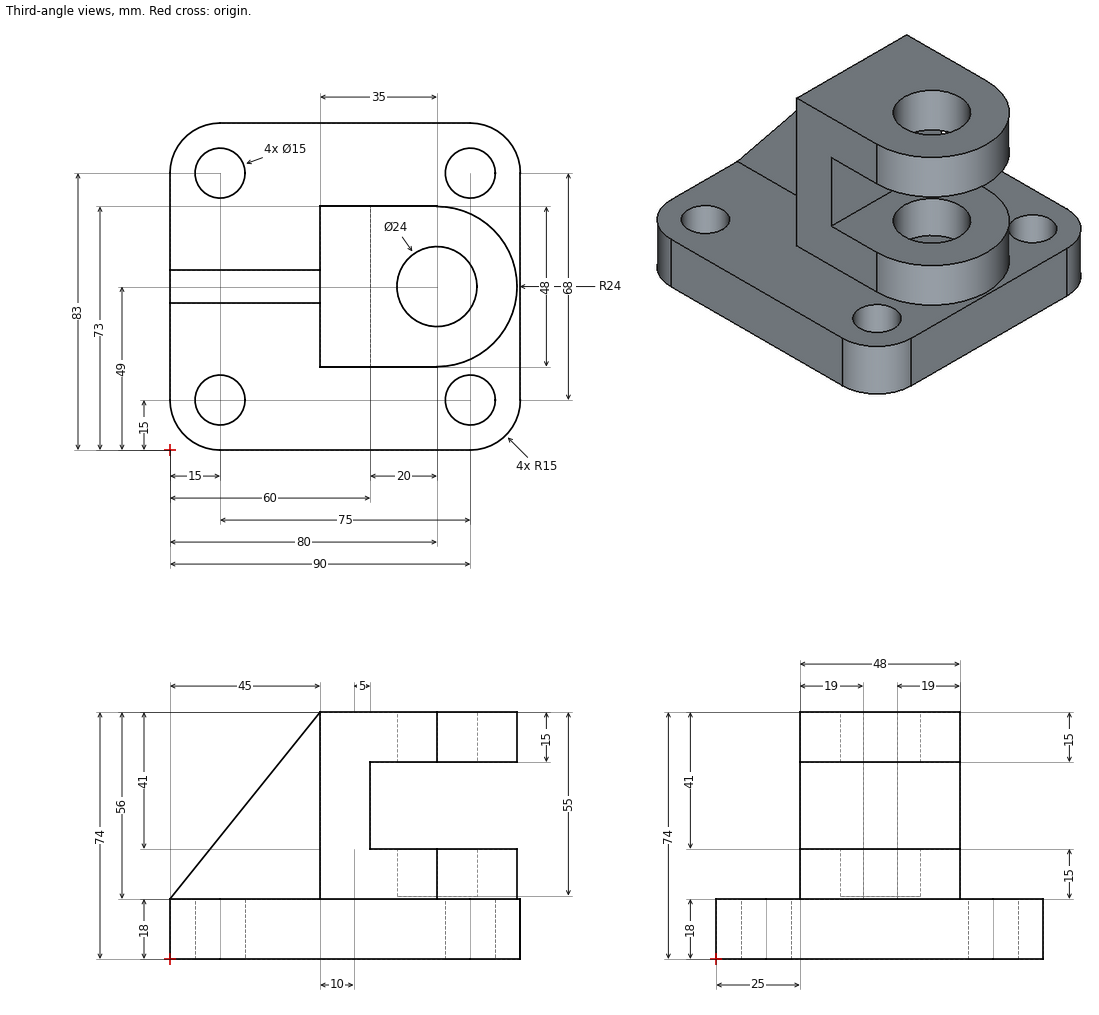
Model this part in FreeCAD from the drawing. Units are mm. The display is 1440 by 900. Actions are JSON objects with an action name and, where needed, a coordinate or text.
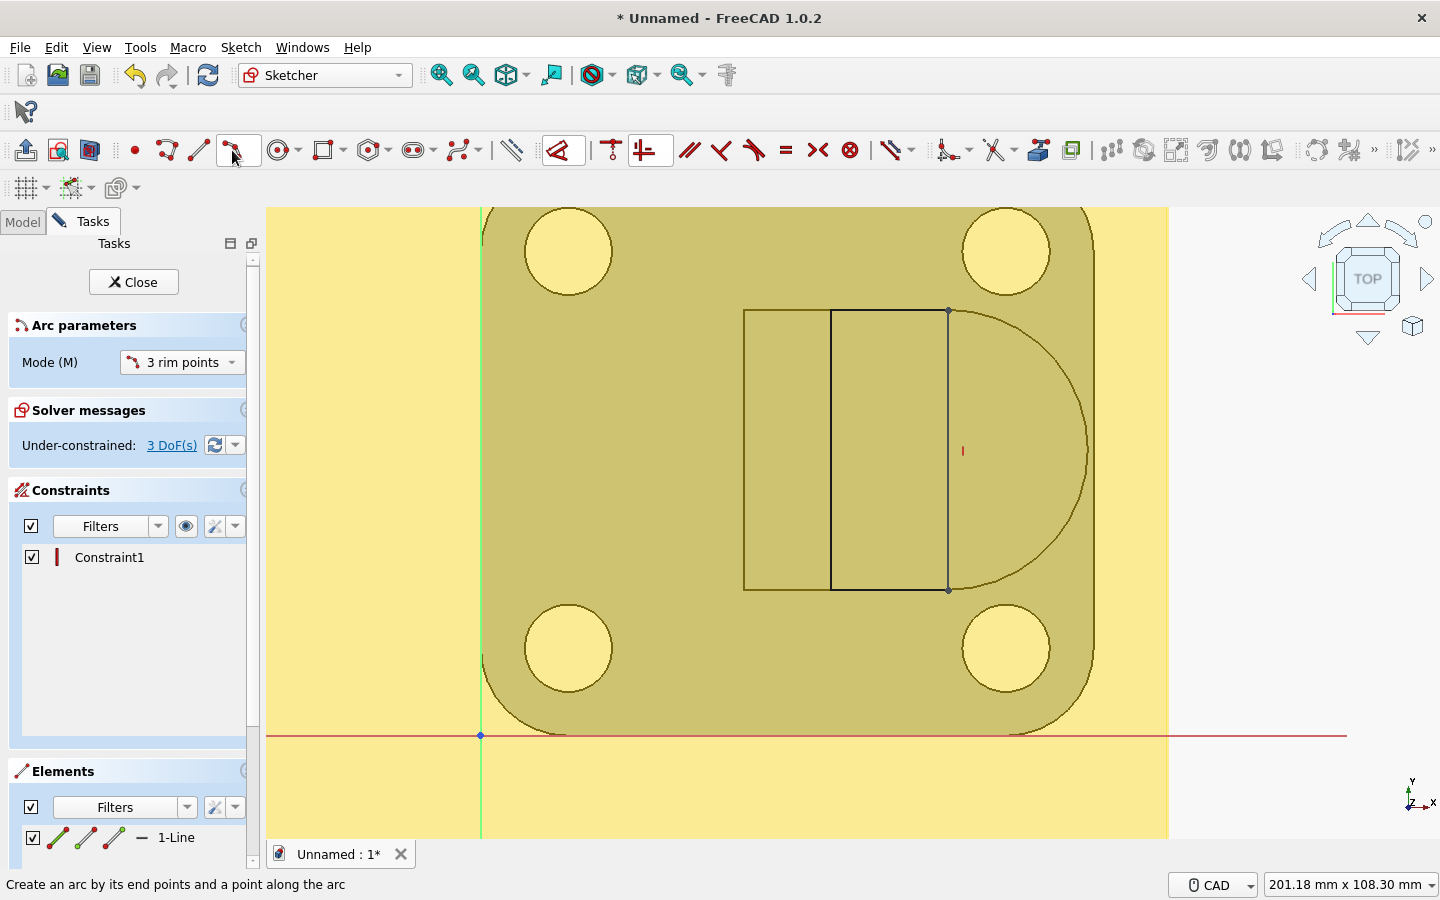
{"action": "left_click", "coordinate": [948, 591]}
{"action": "left_click", "coordinate": [948, 311]}
{"action": "left_click", "coordinate": [1088, 450]}
{"action": "key", "text": "Escape"}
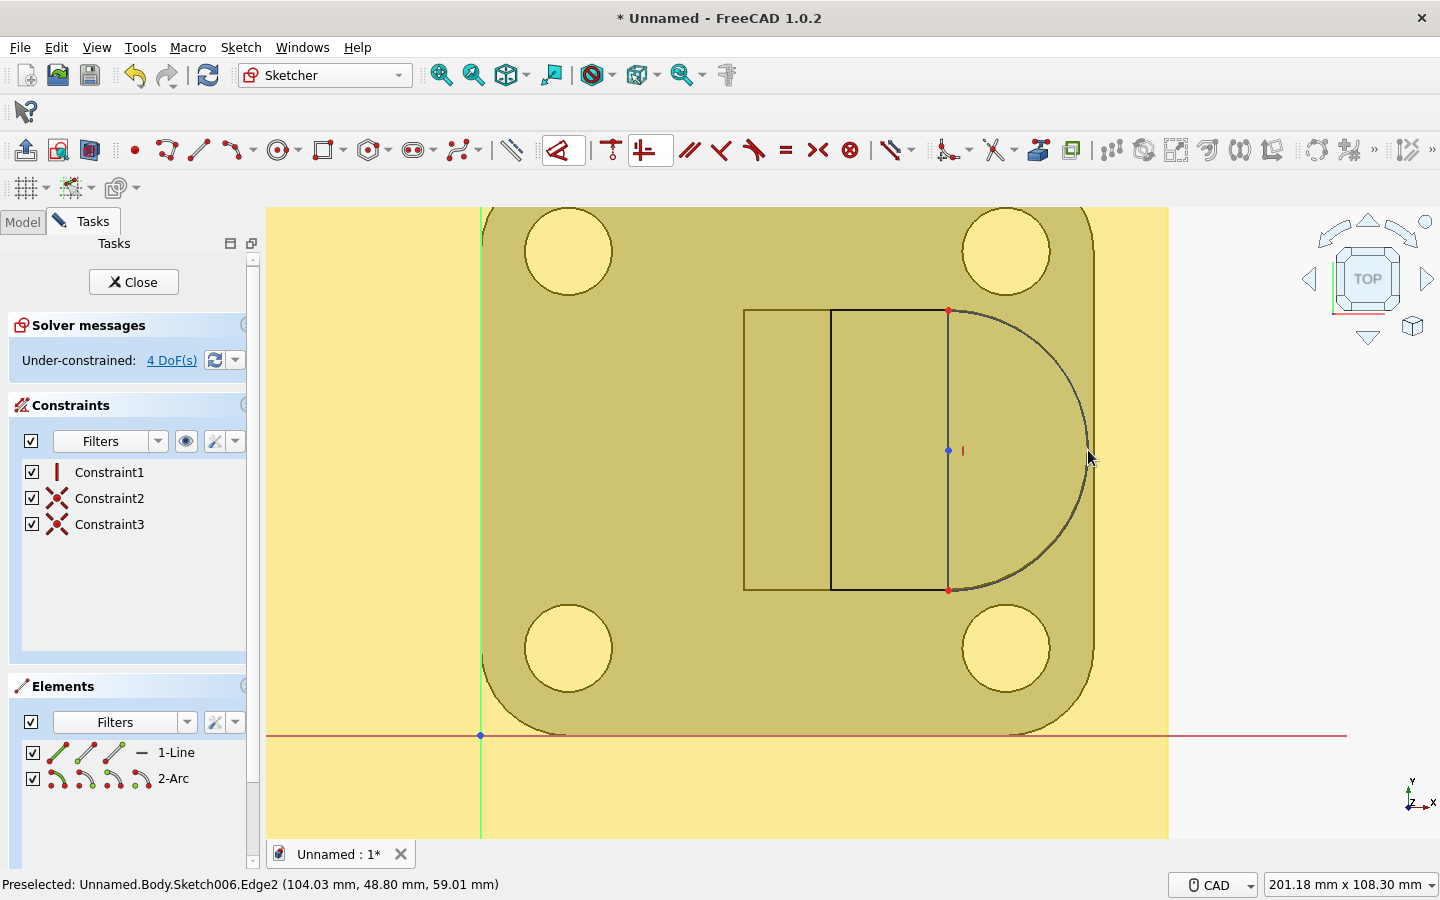
{"action": "left_click", "coordinate": [1061, 533]}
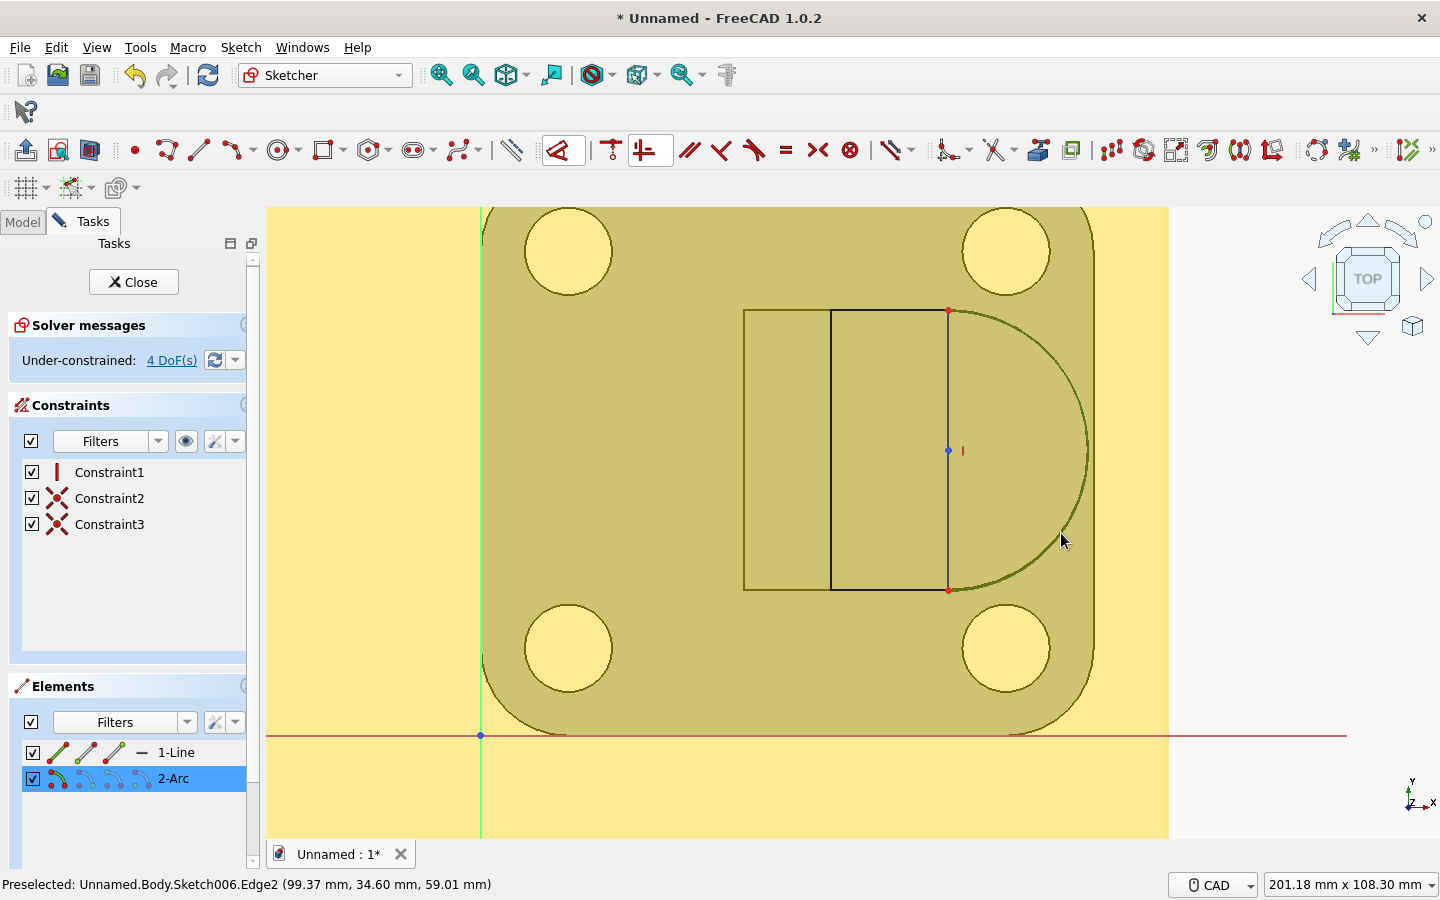
{"action": "left_click", "coordinate": [580, 150]}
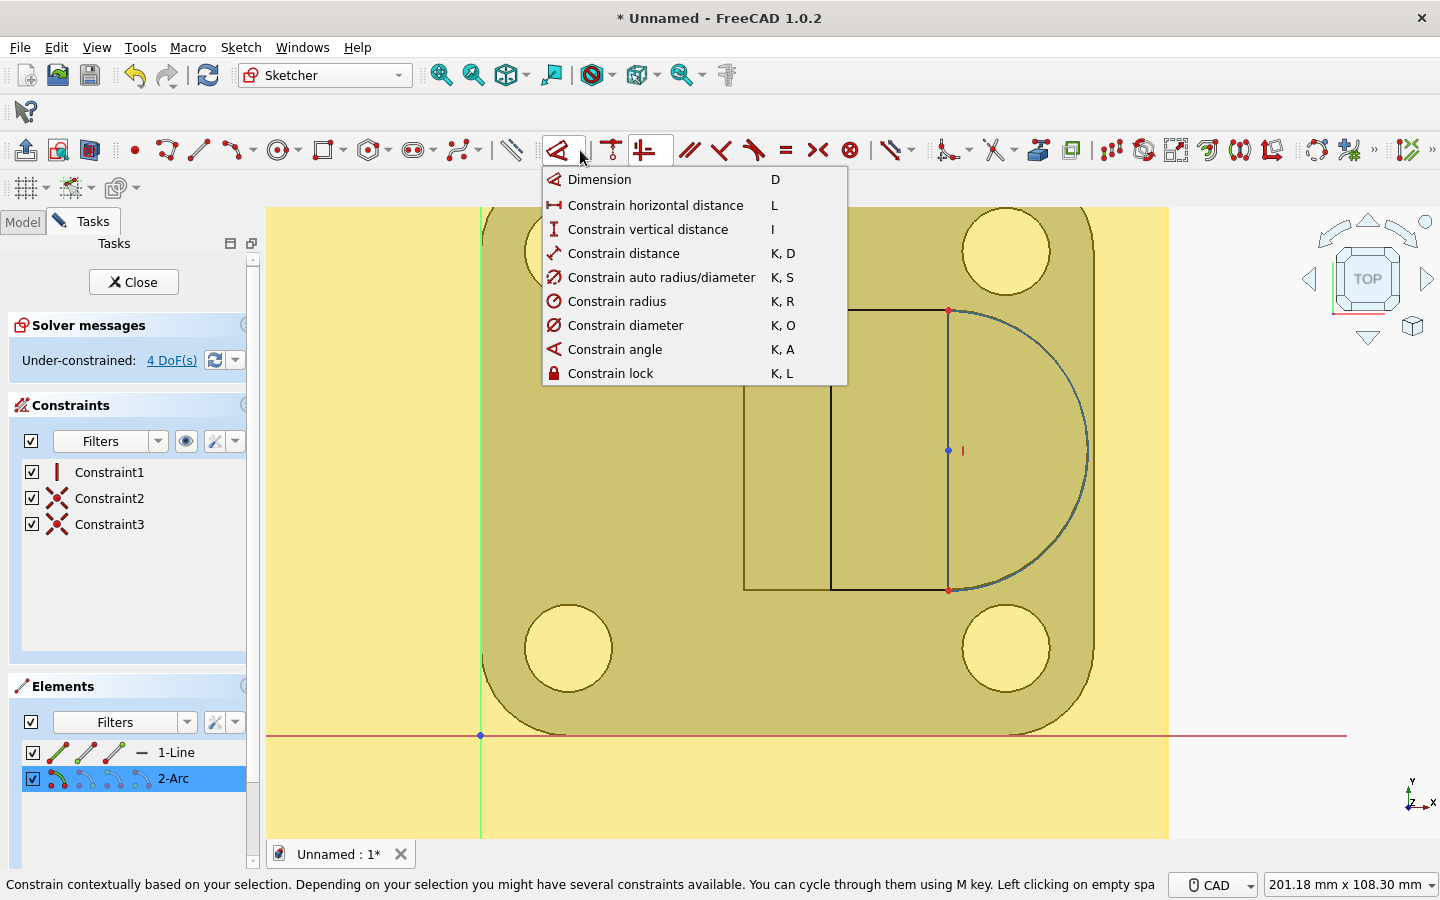
{"action": "left_click", "coordinate": [695, 301]}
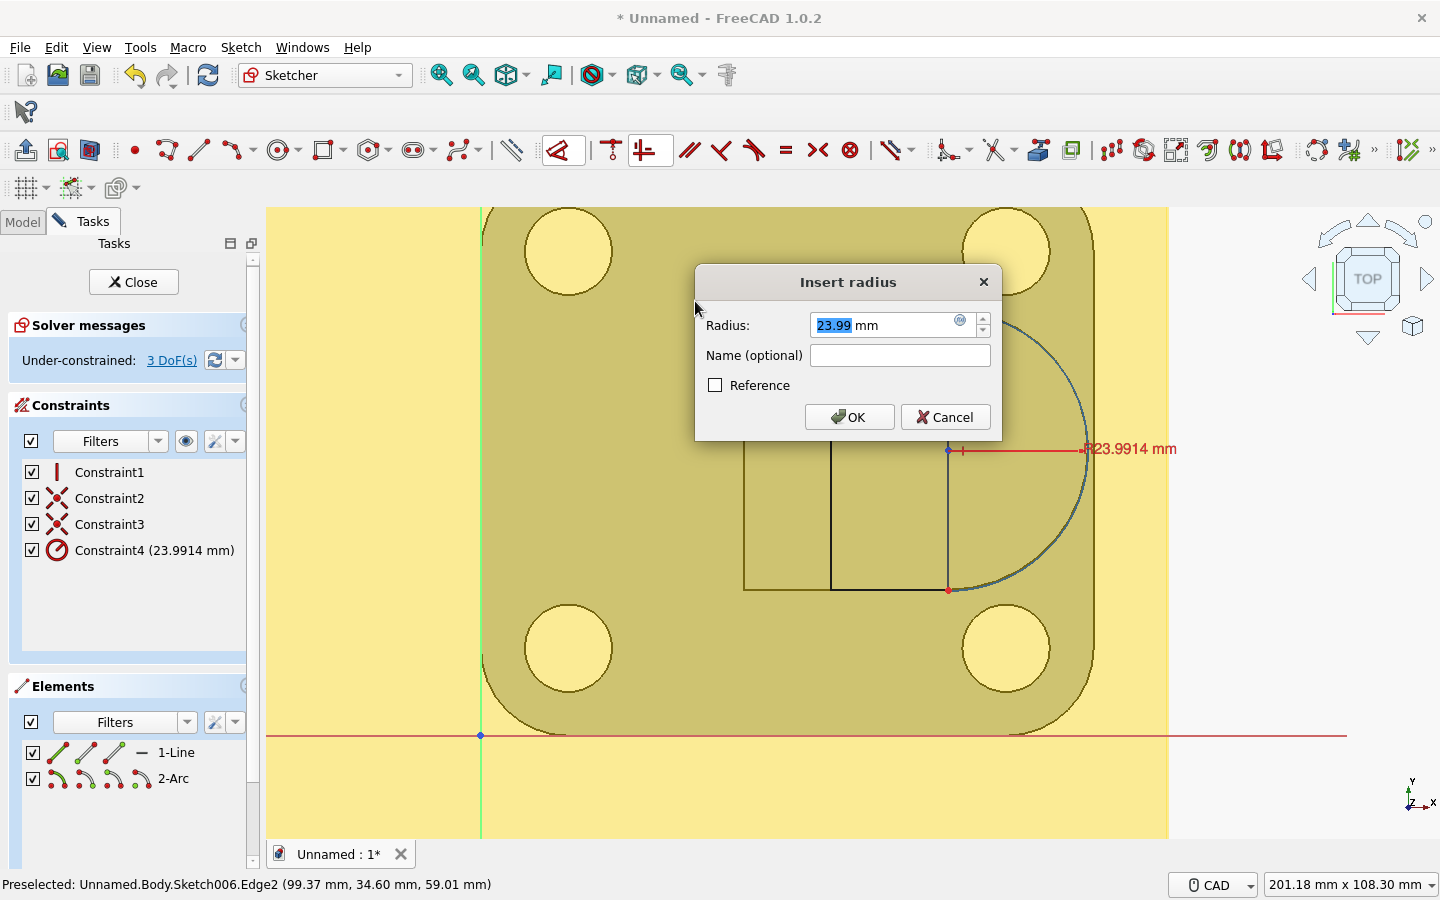
{"action": "type", "text": "24"}
{"action": "key", "text": "Return"}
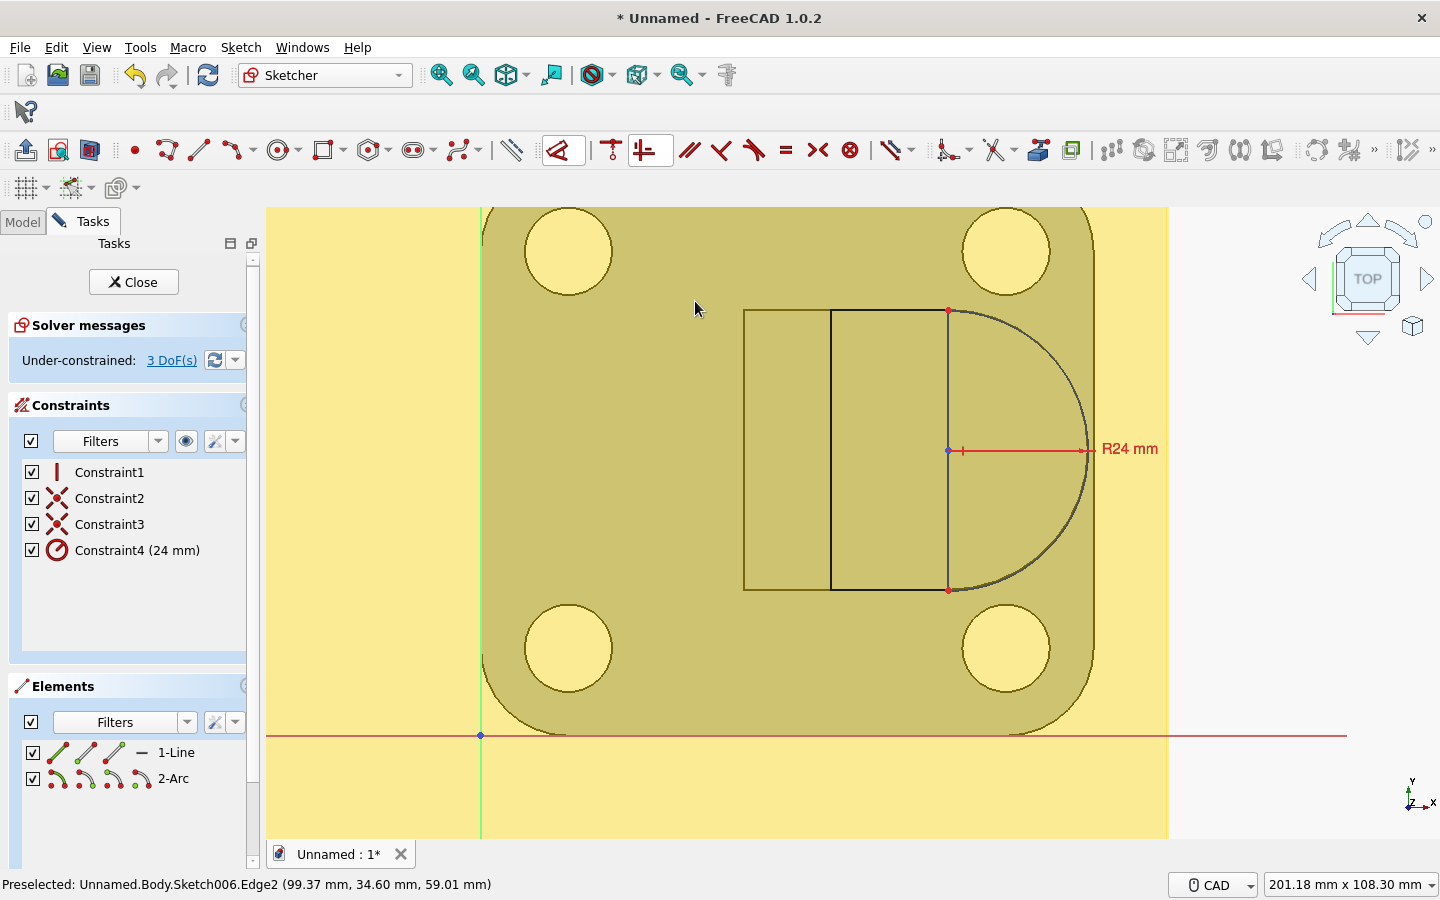
{"action": "left_click", "coordinate": [948, 311]}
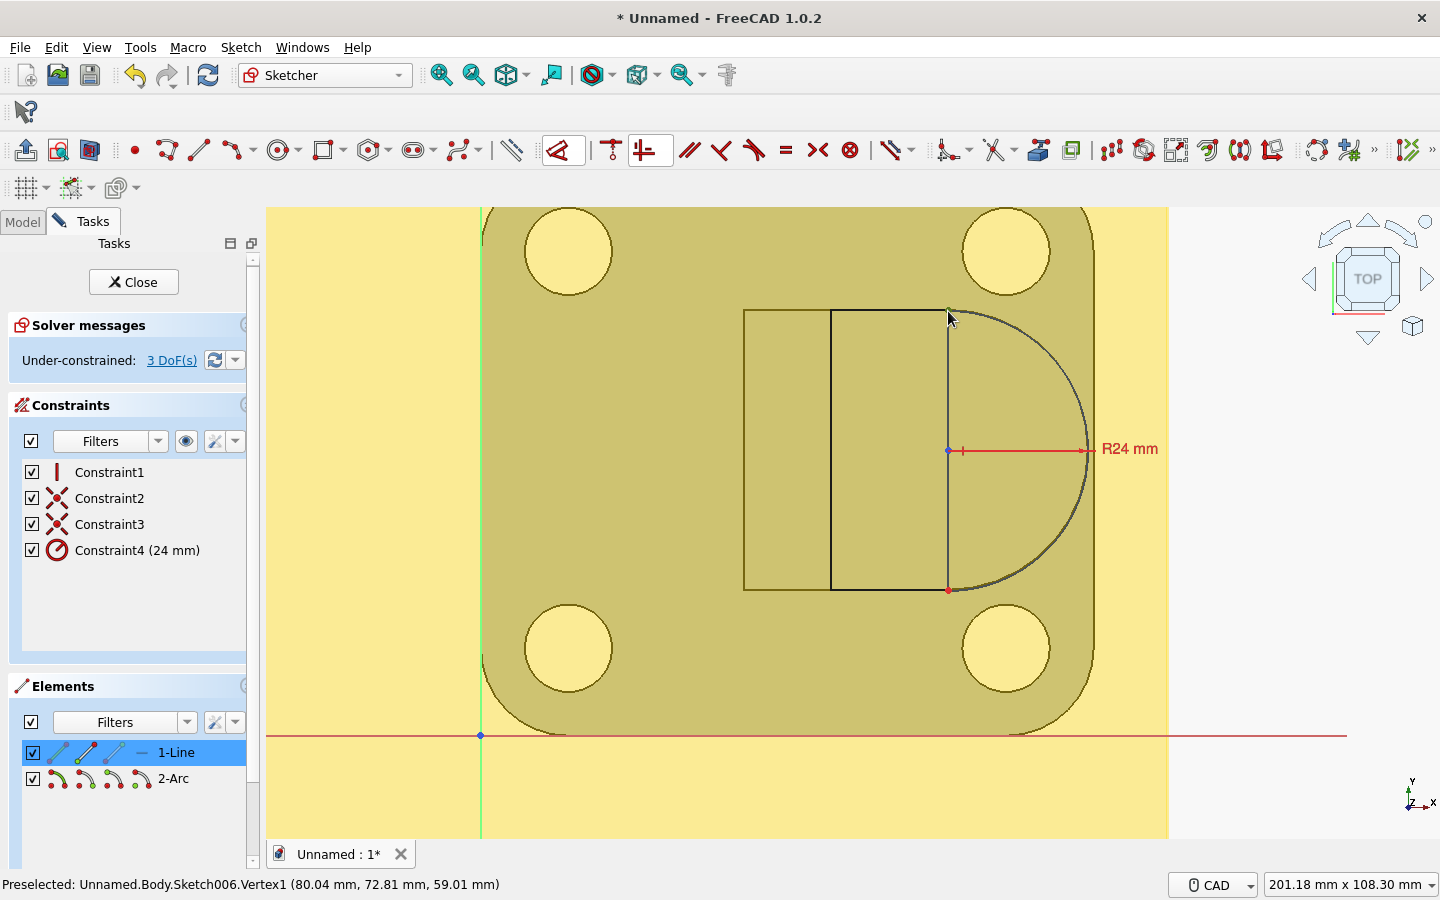
{"action": "key", "text": "l"}